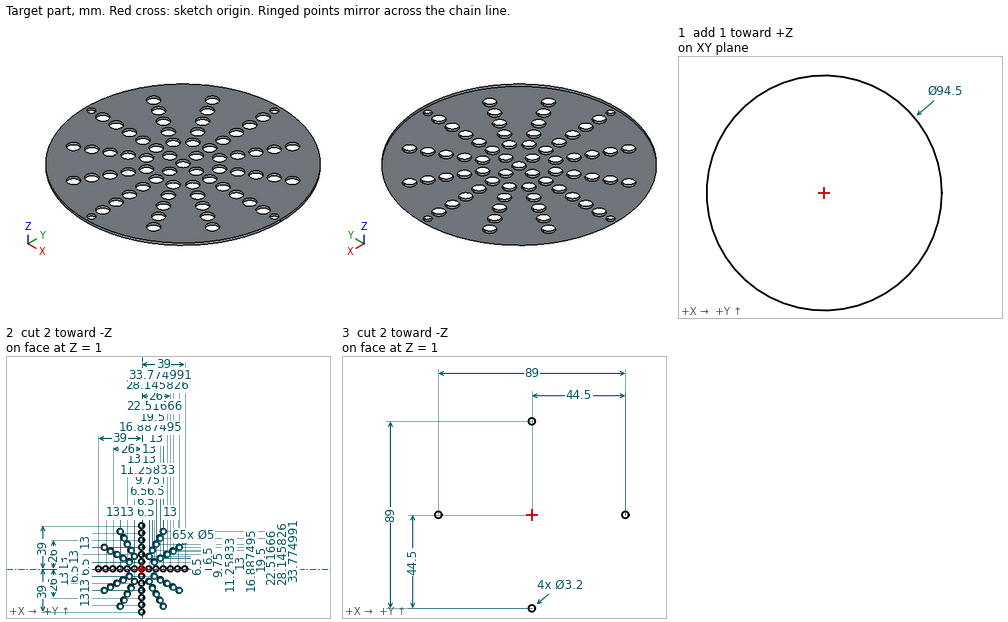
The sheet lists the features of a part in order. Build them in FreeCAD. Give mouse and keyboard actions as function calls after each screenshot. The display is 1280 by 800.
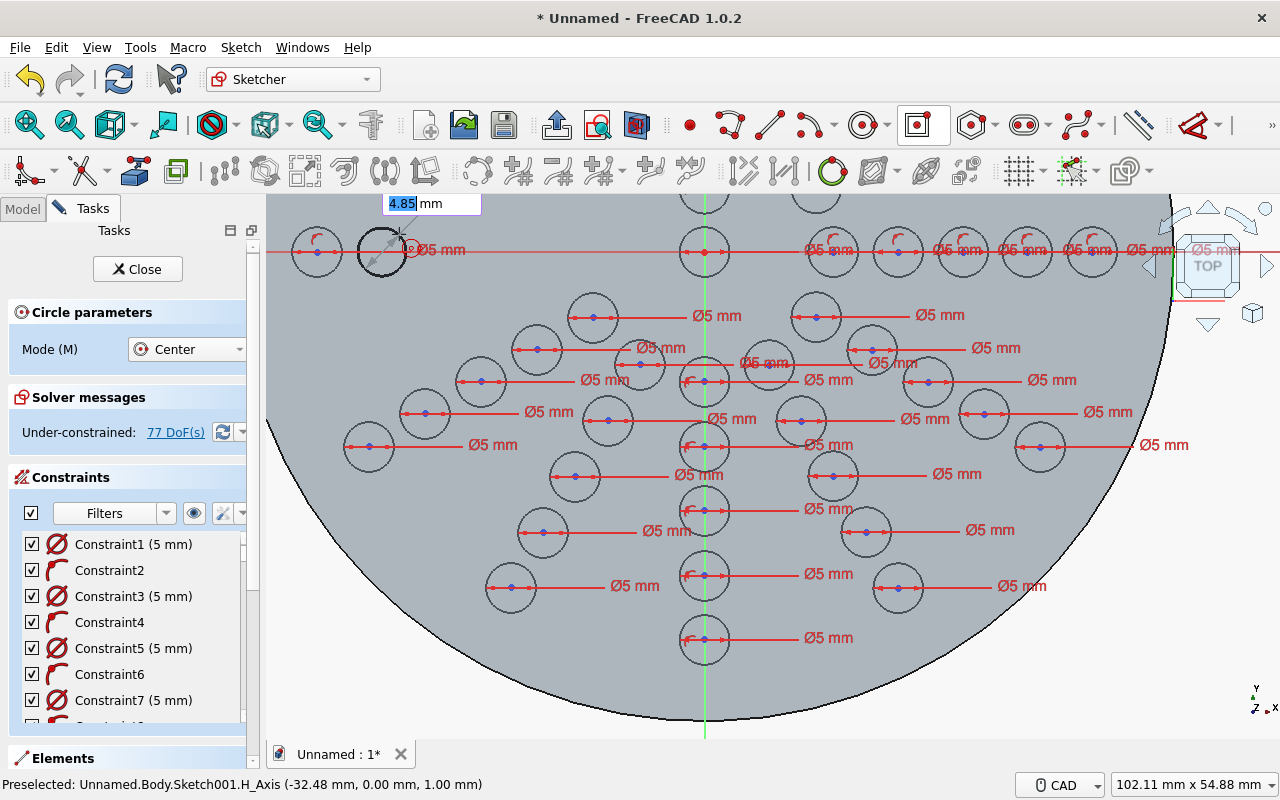
text(5)
key(Return)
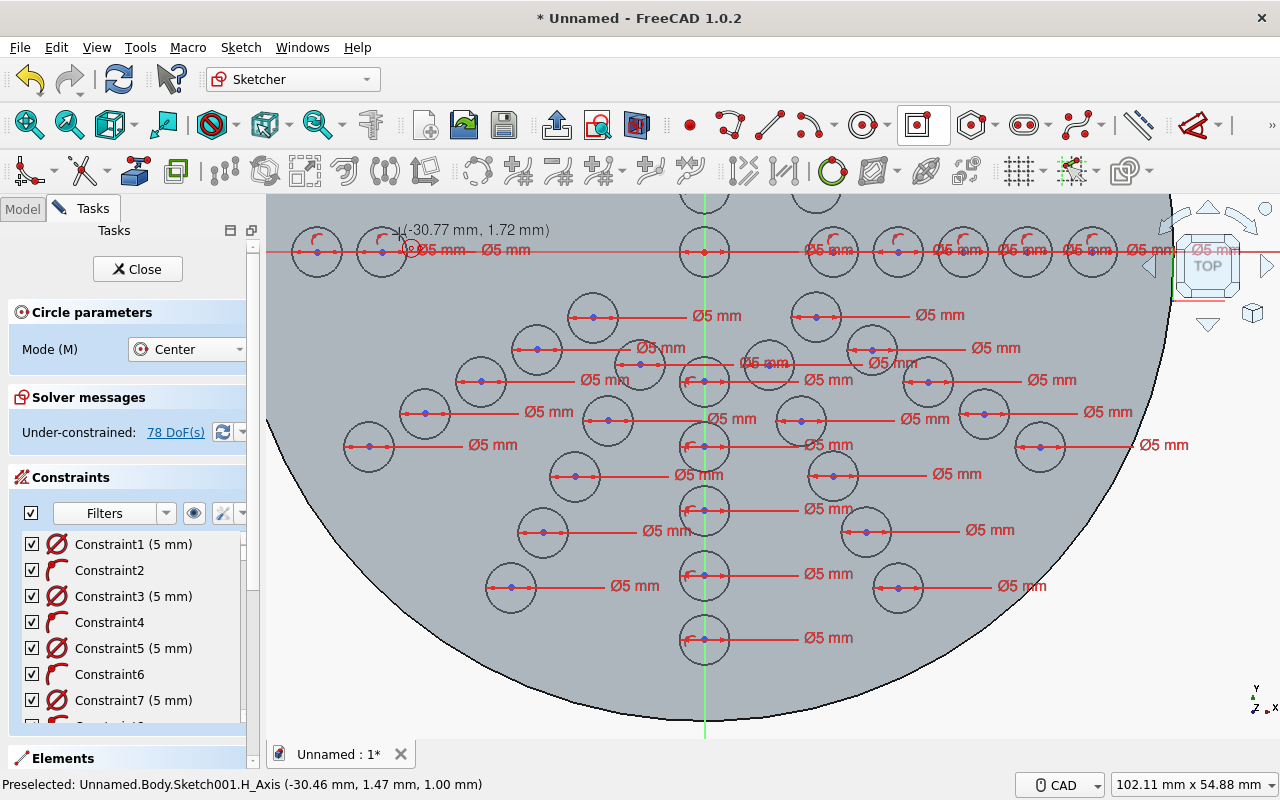
click(446, 252)
move(464, 234)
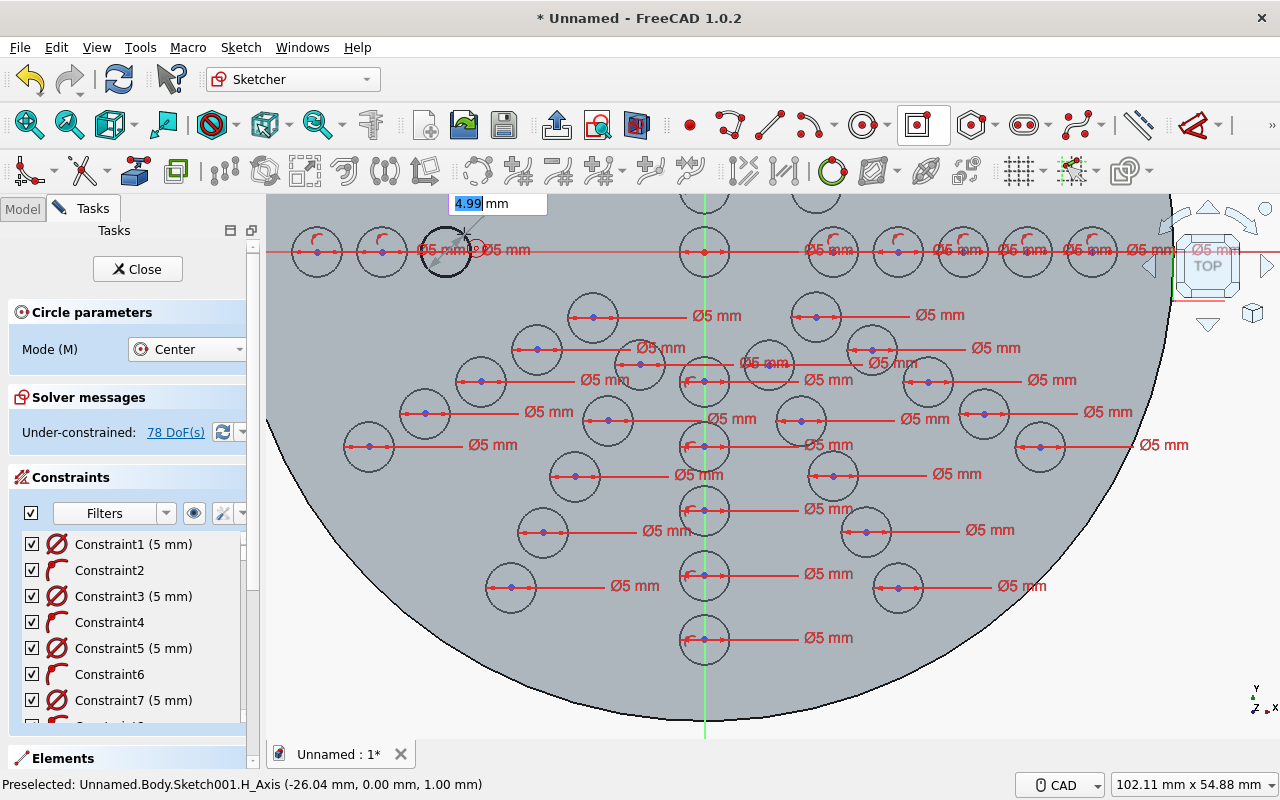
text(5)
key(Return)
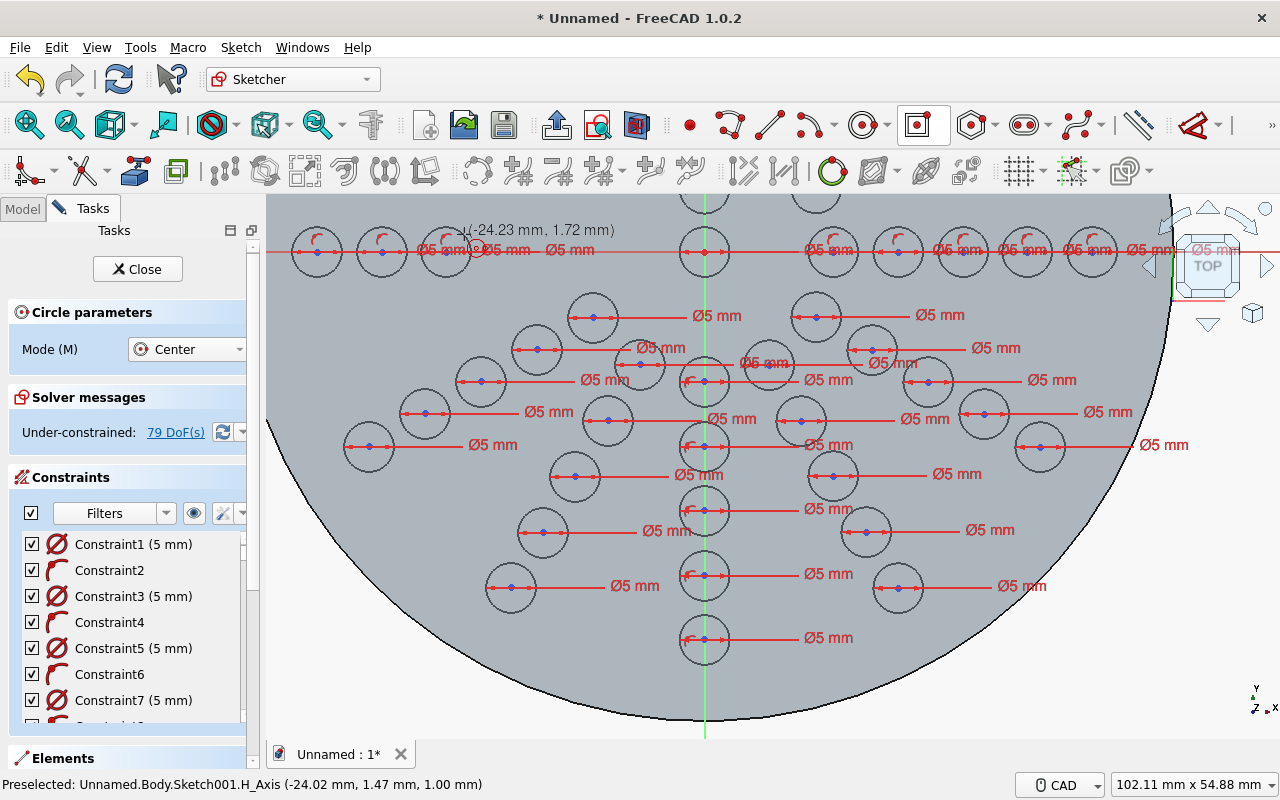
click(511, 252)
move(528, 234)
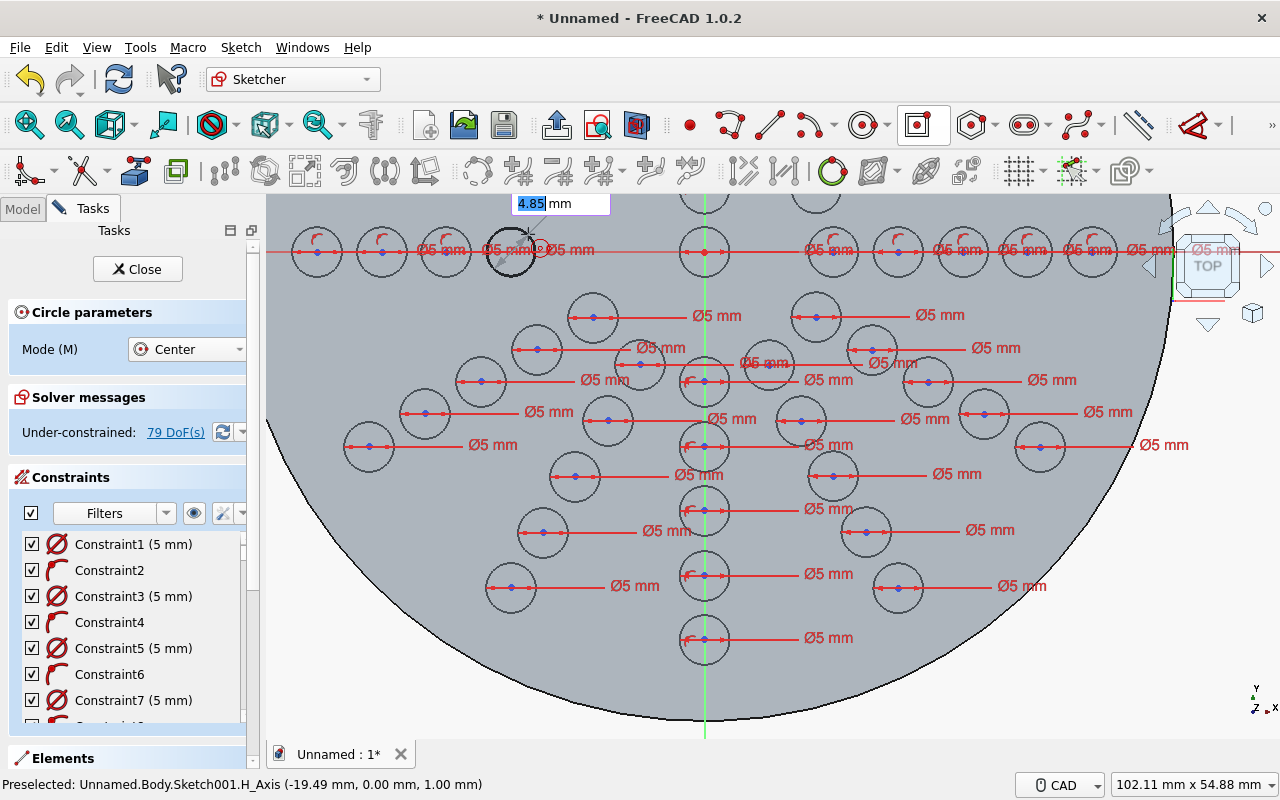
text(5)
key(Return)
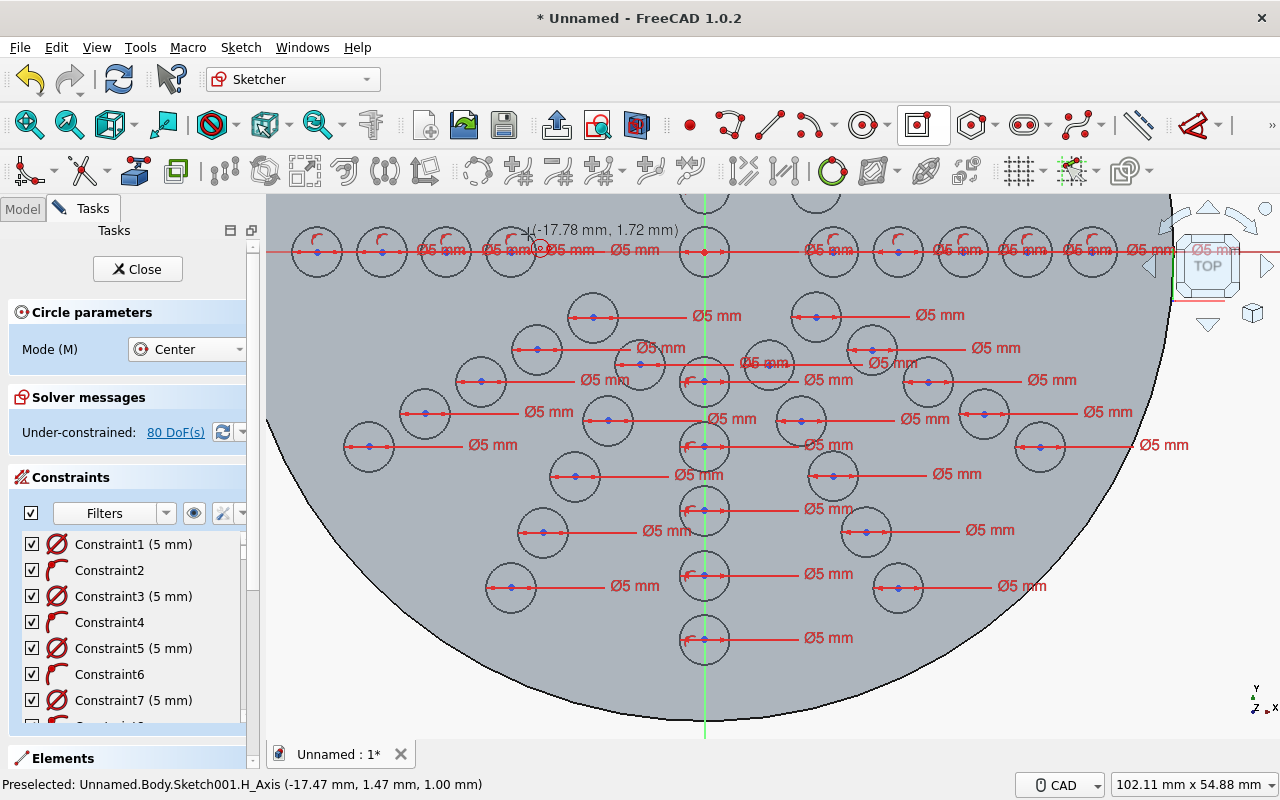
click(575, 252)
move(593, 234)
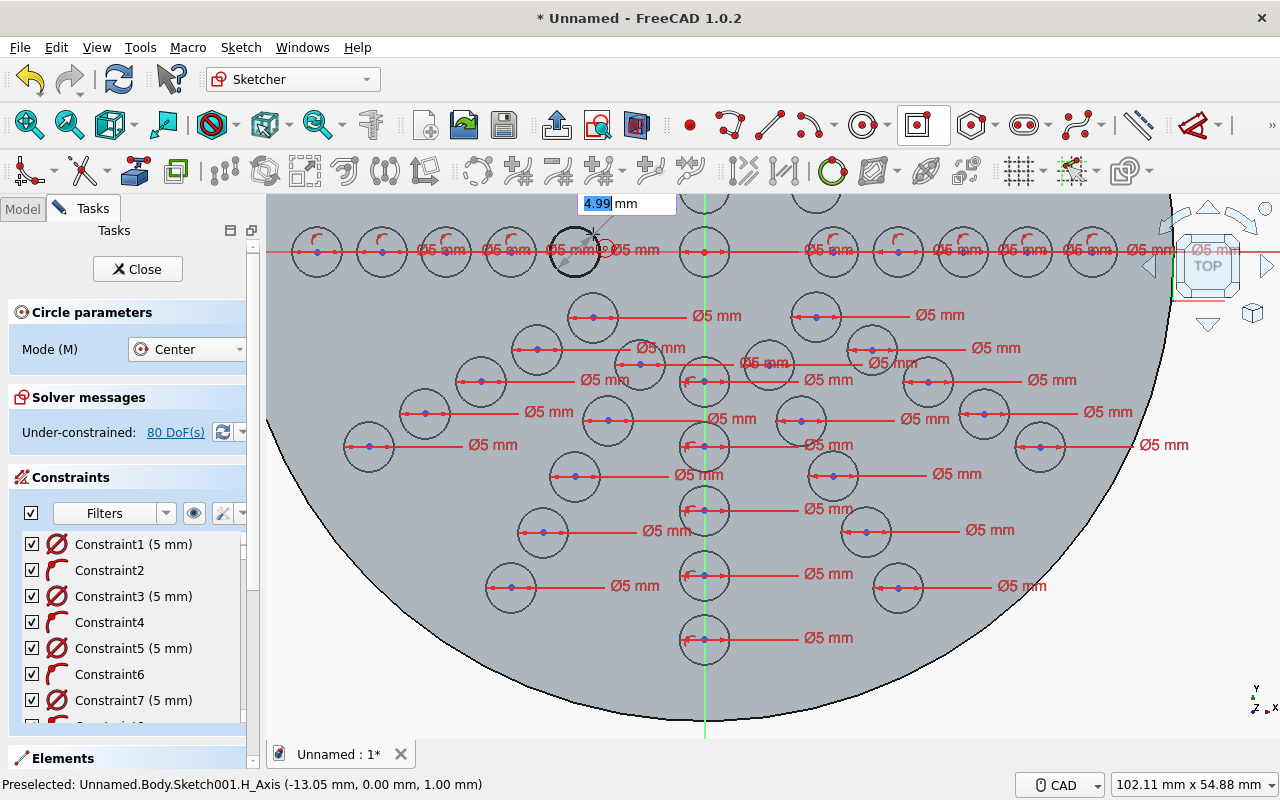
text(5)
key(Return)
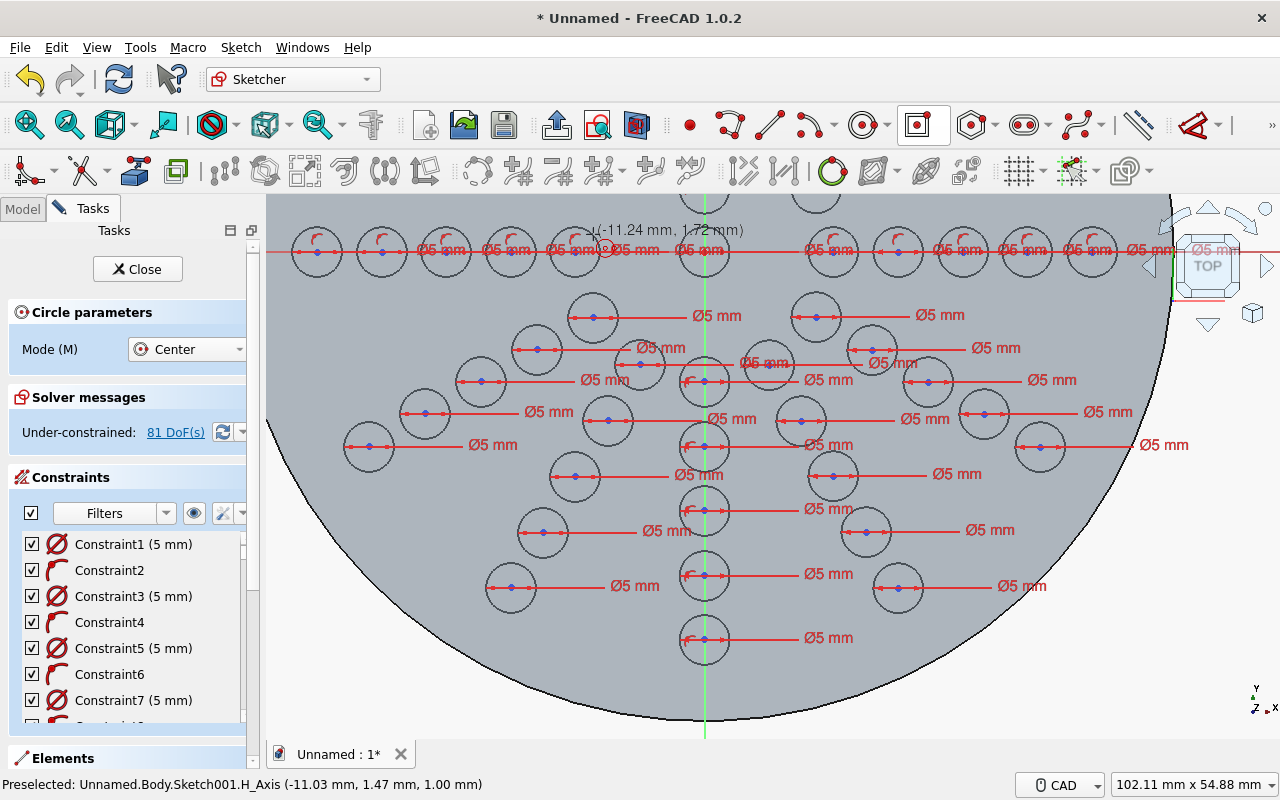
scroll(704, 641, down, 4)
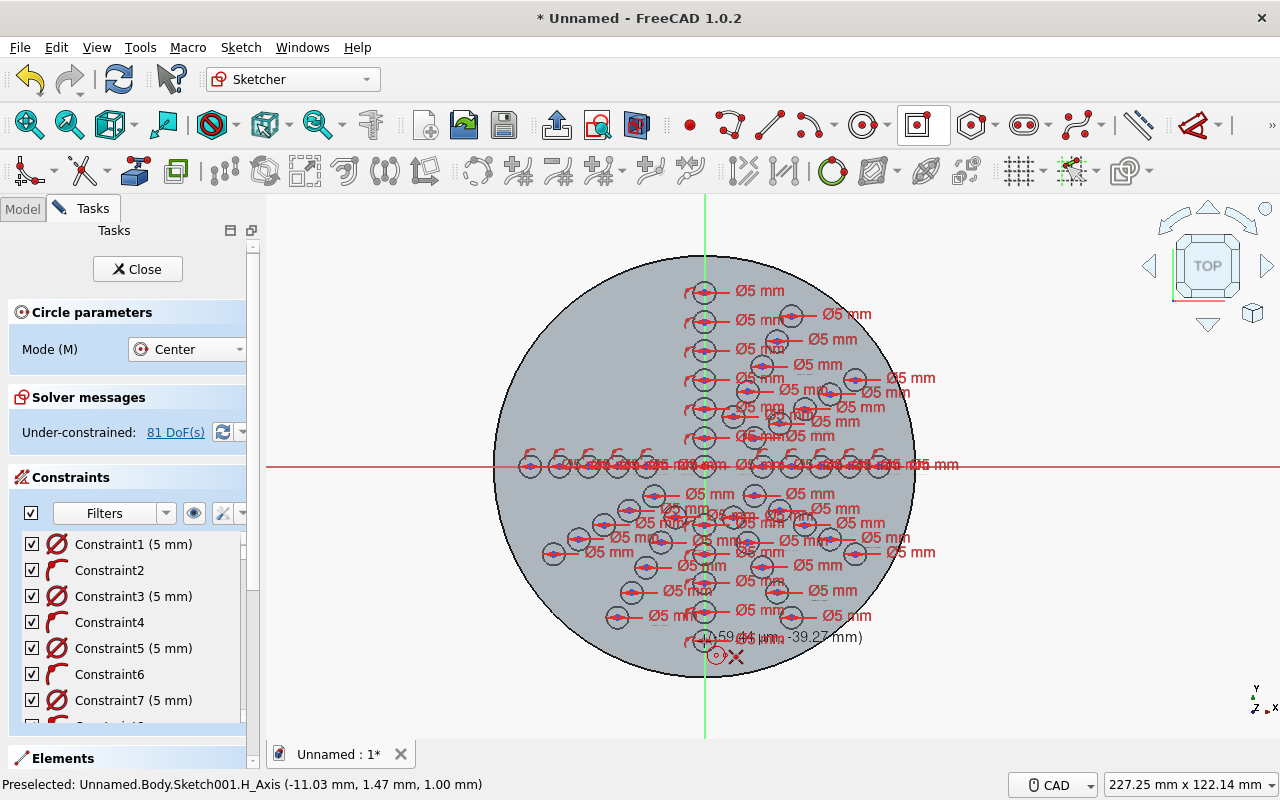
scroll(554, 380, up, 4)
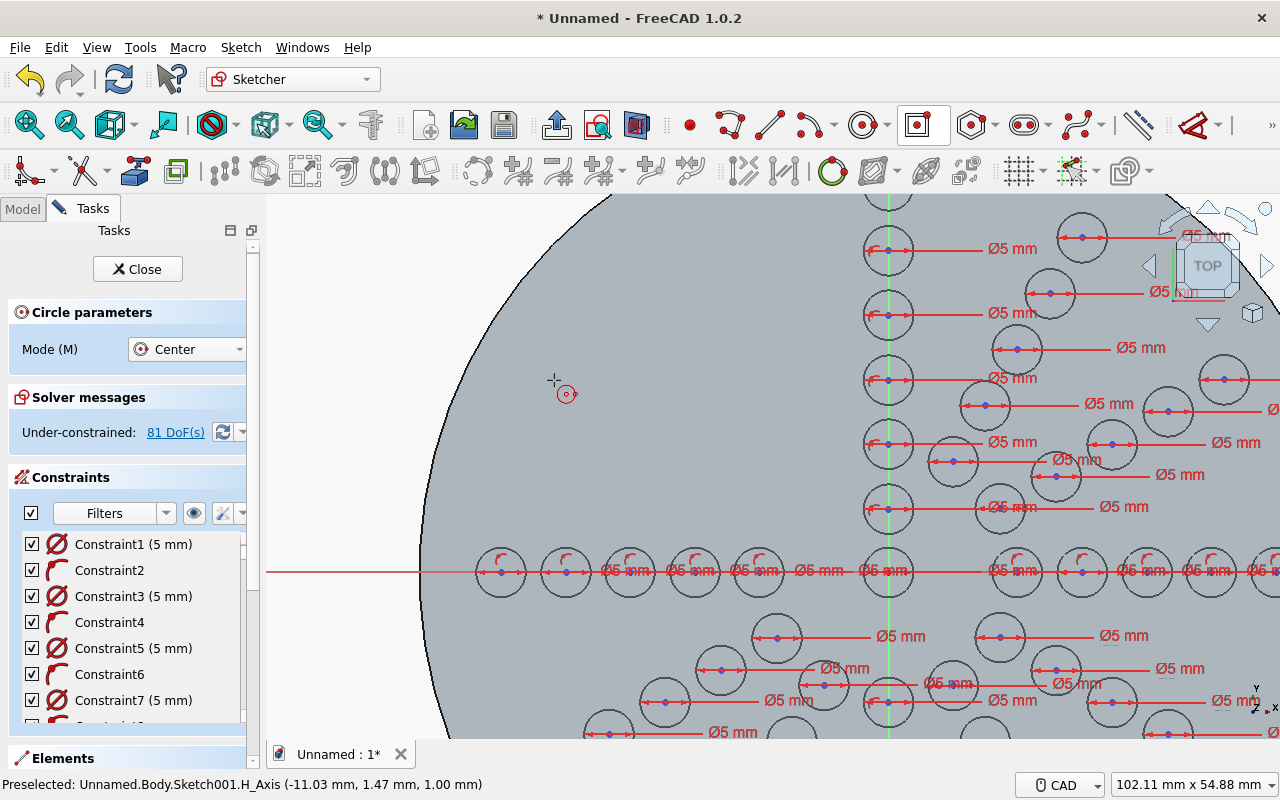
click(553, 379)
move(571, 361)